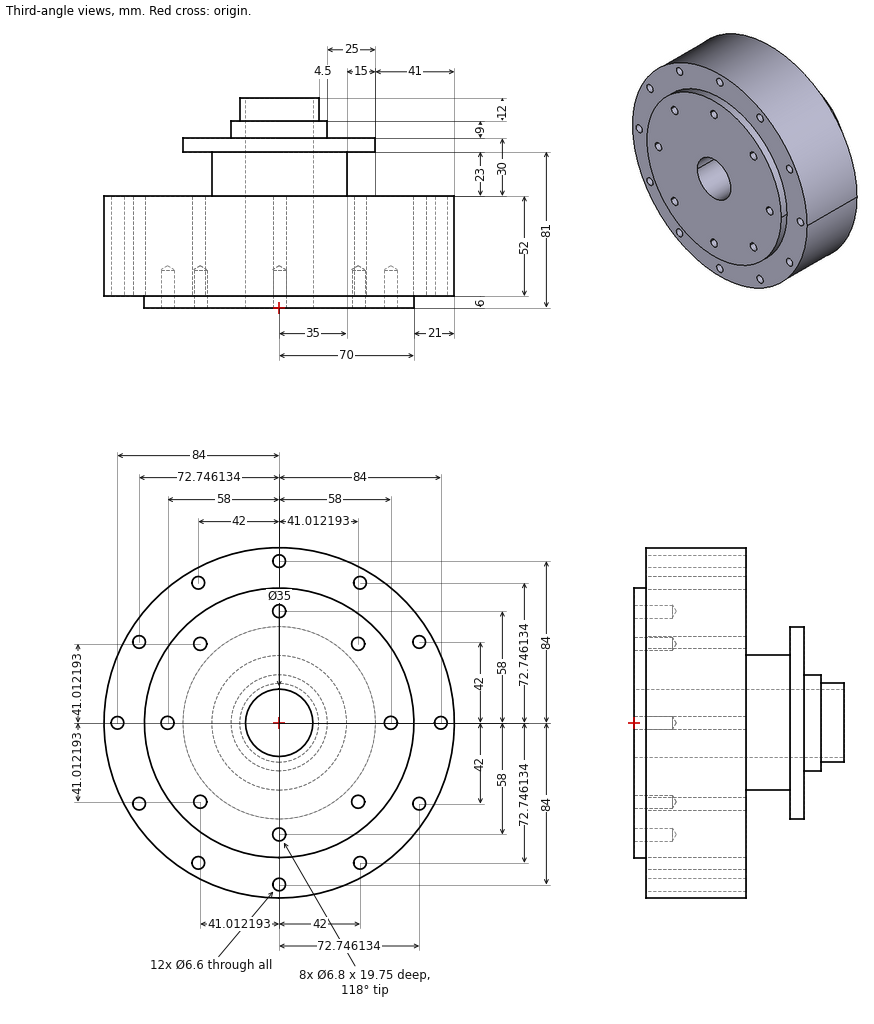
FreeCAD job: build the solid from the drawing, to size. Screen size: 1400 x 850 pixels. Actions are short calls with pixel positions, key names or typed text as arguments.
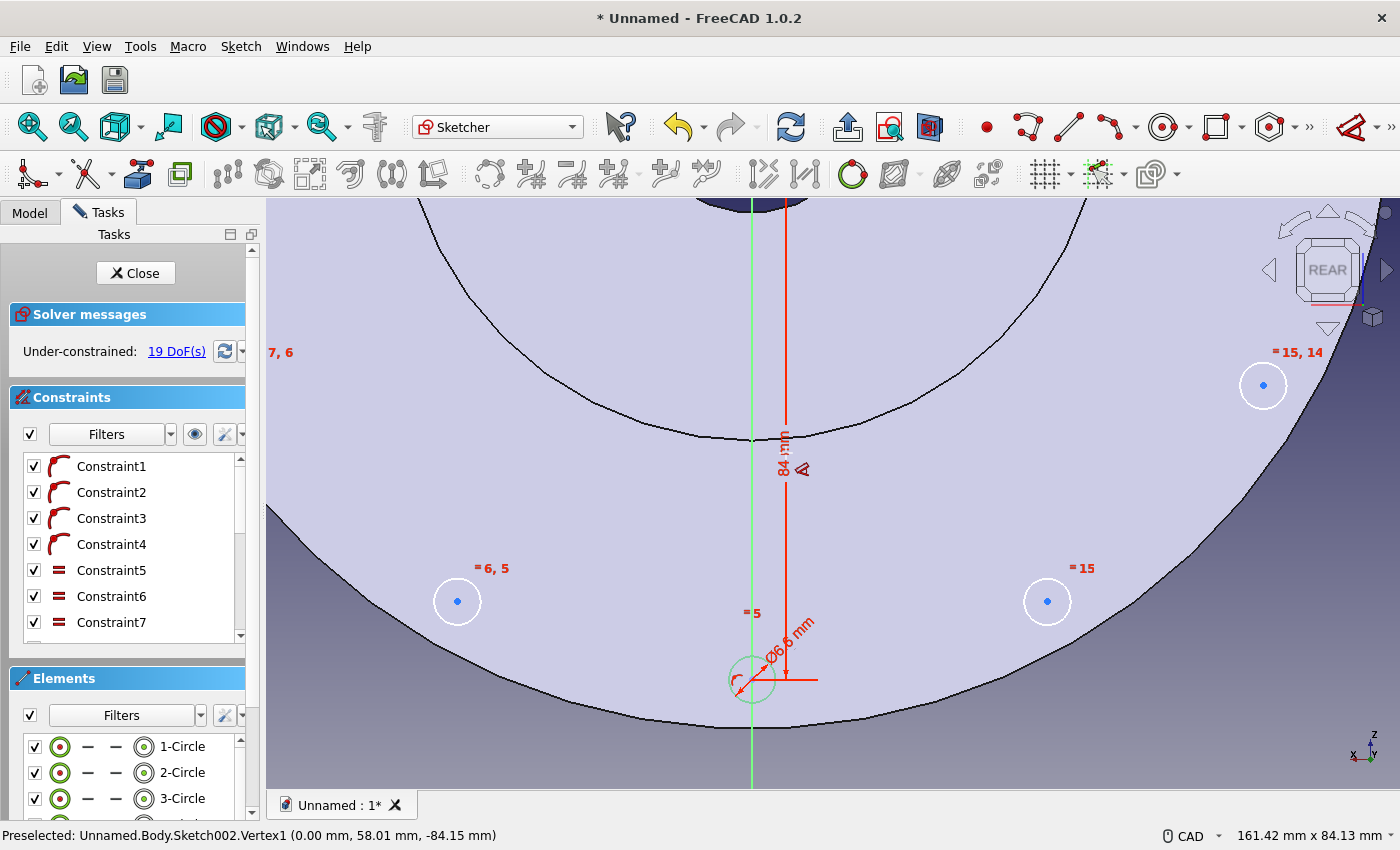
click(457, 602)
click(605, 636)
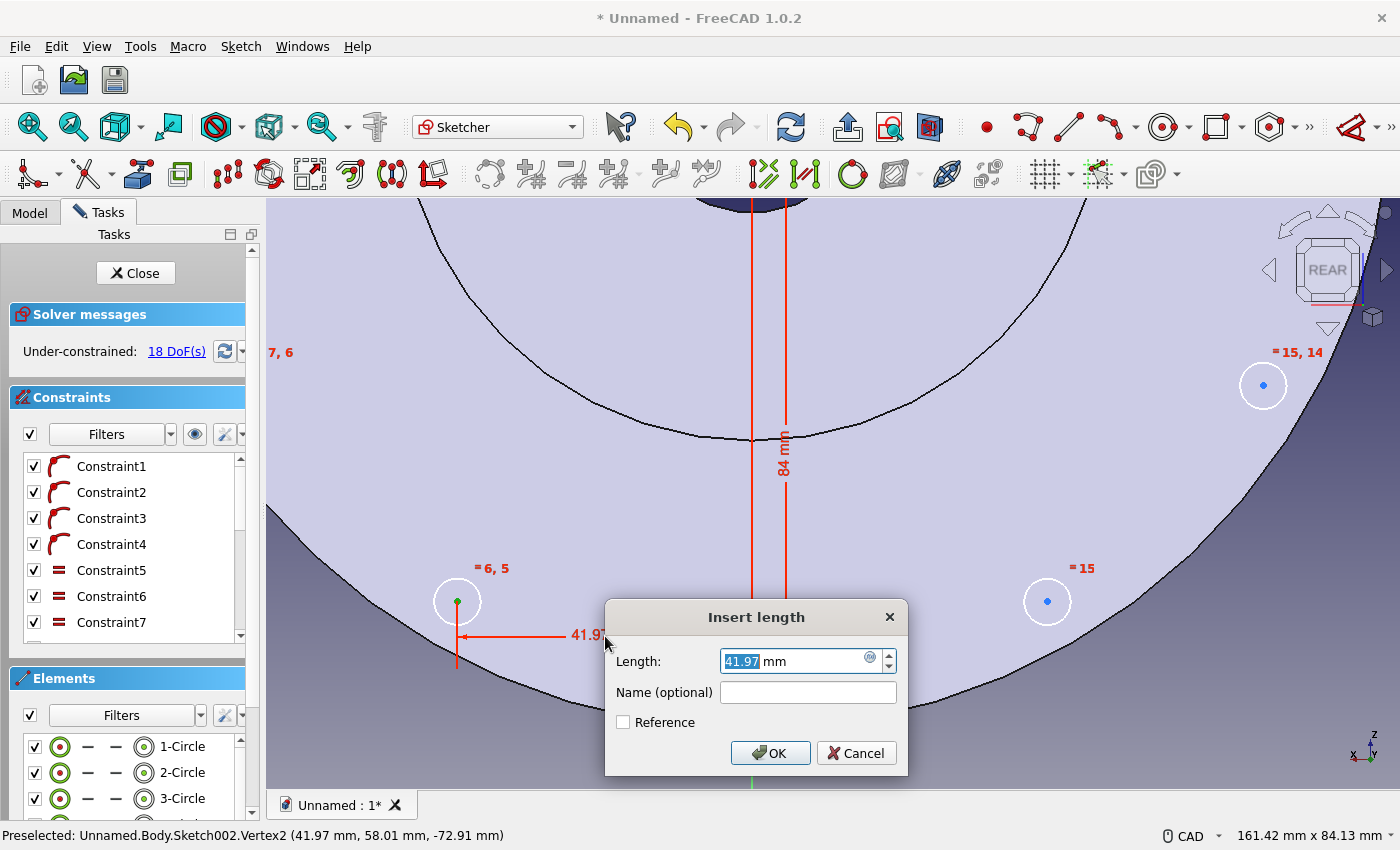
text(42)
key(Return)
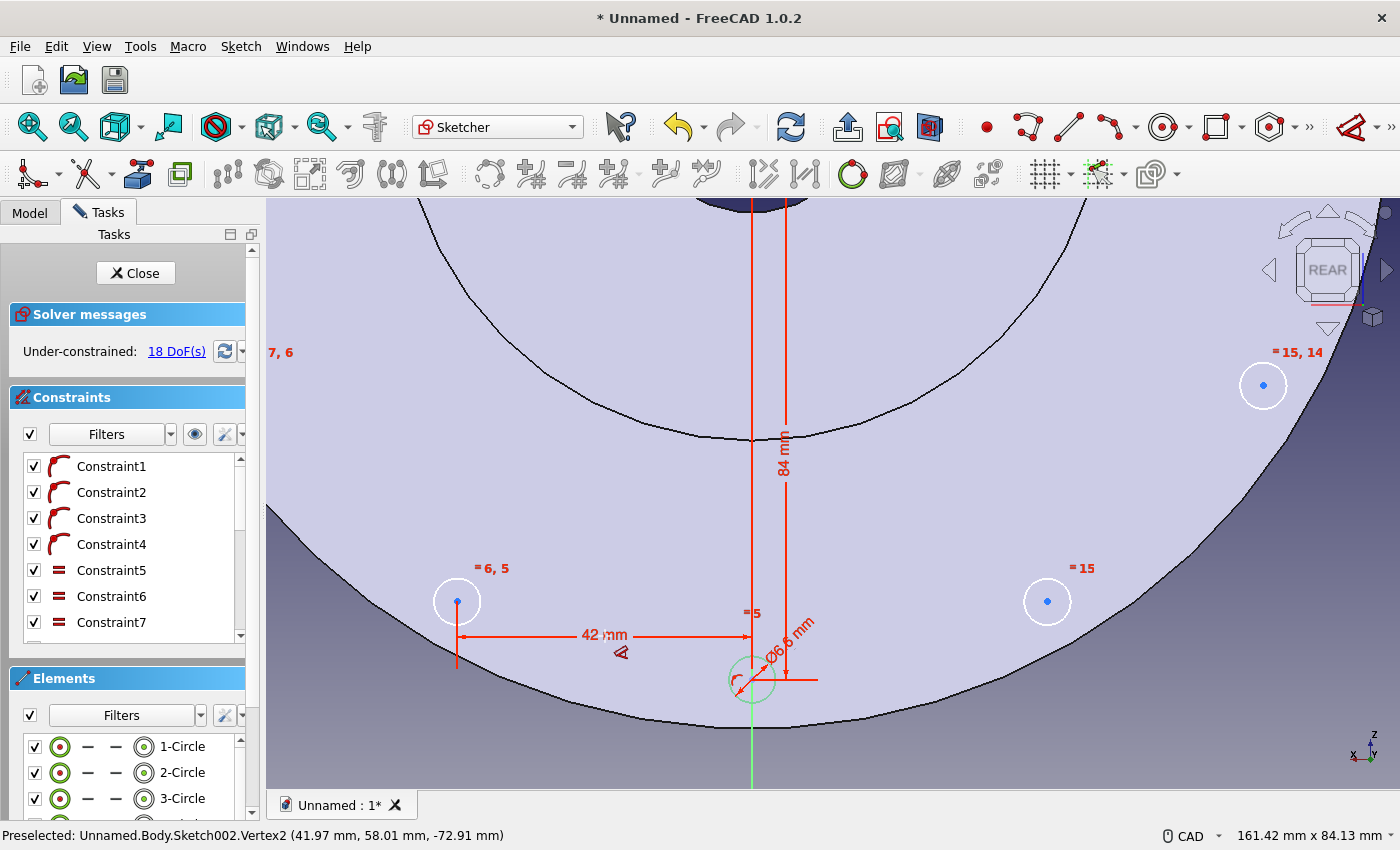
scroll(770, 668, down, 6)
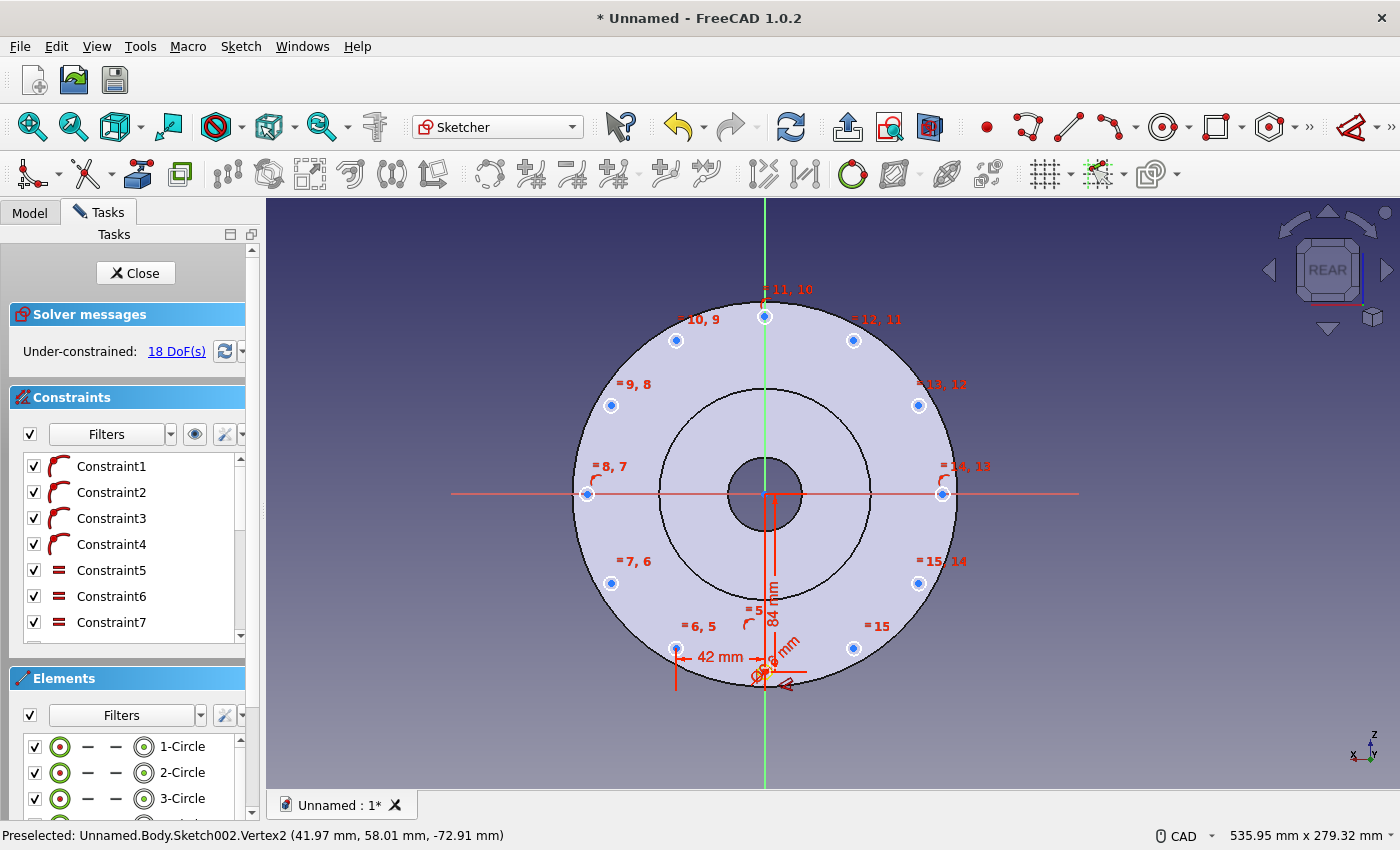
click(611, 584)
click(577, 539)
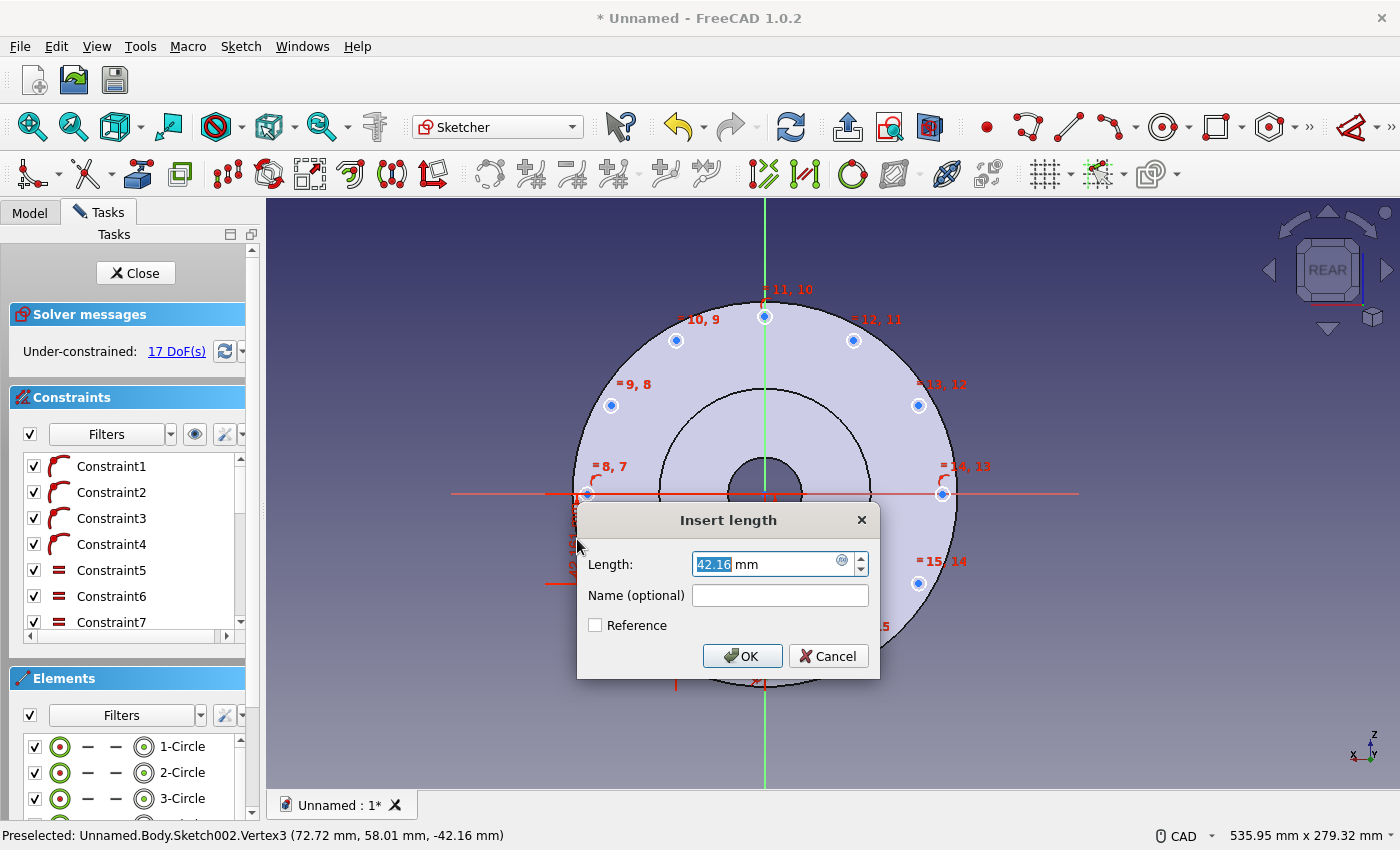
text(42)
key(Return)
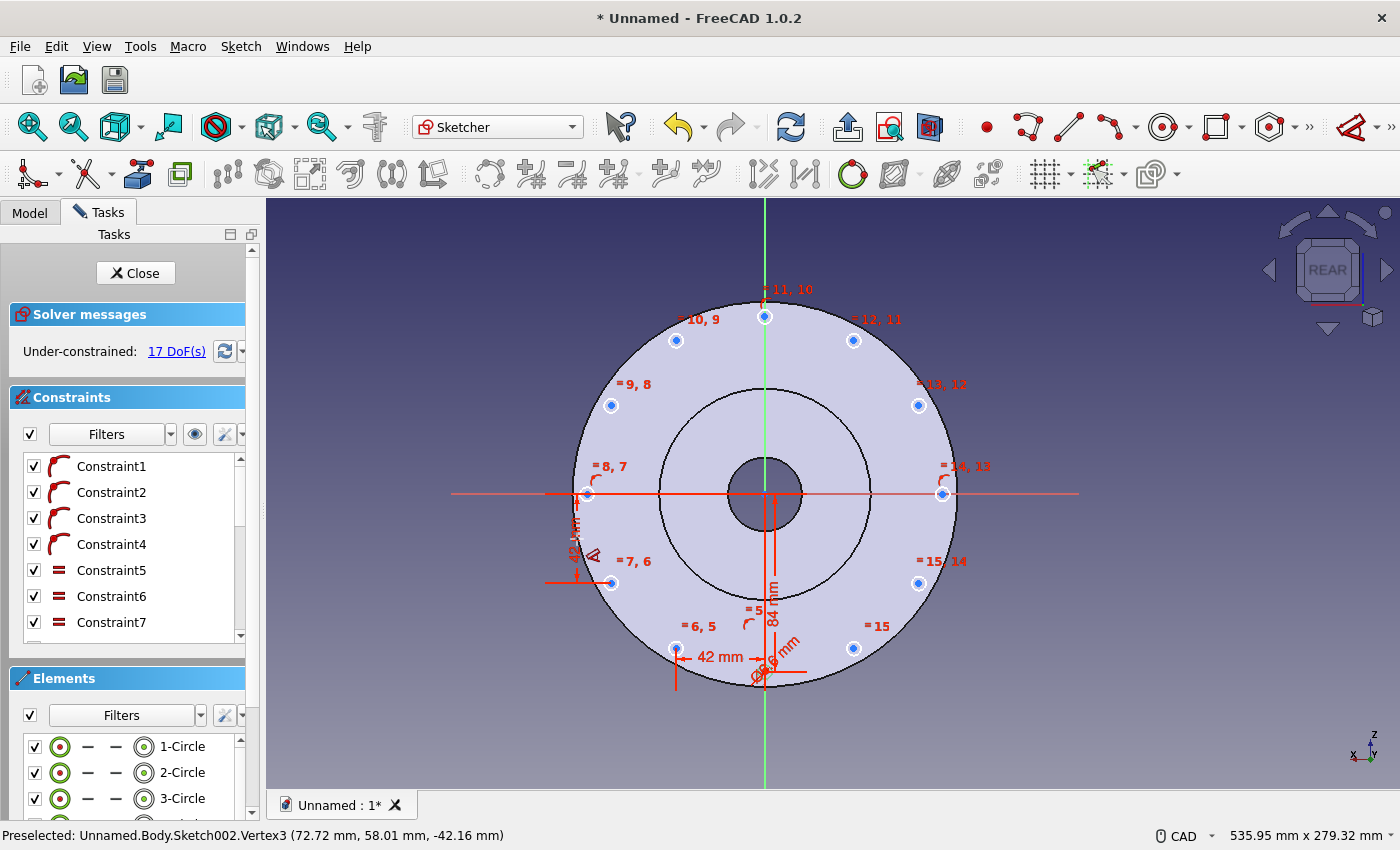
click(587, 494)
click(676, 528)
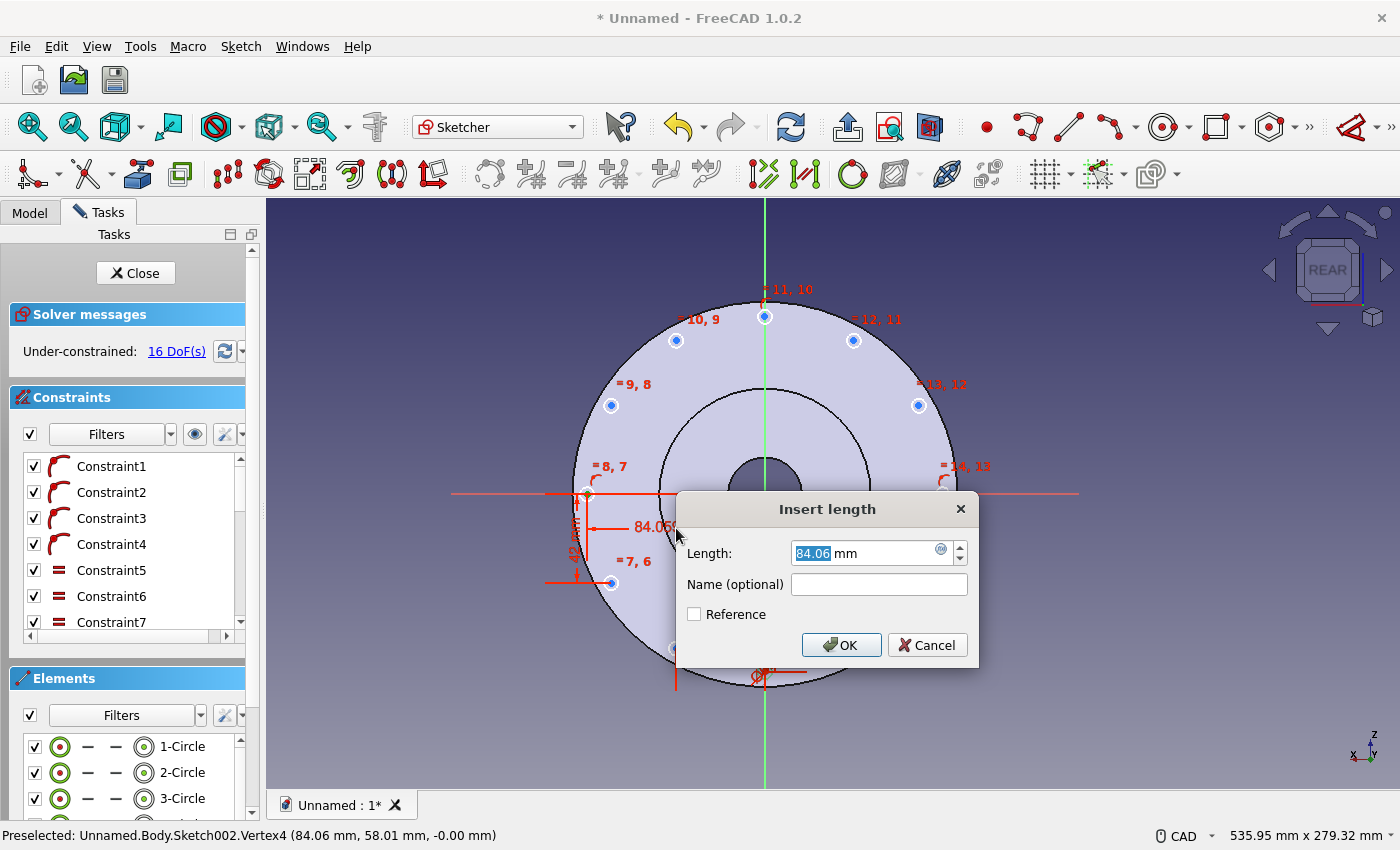
text(84)
key(Return)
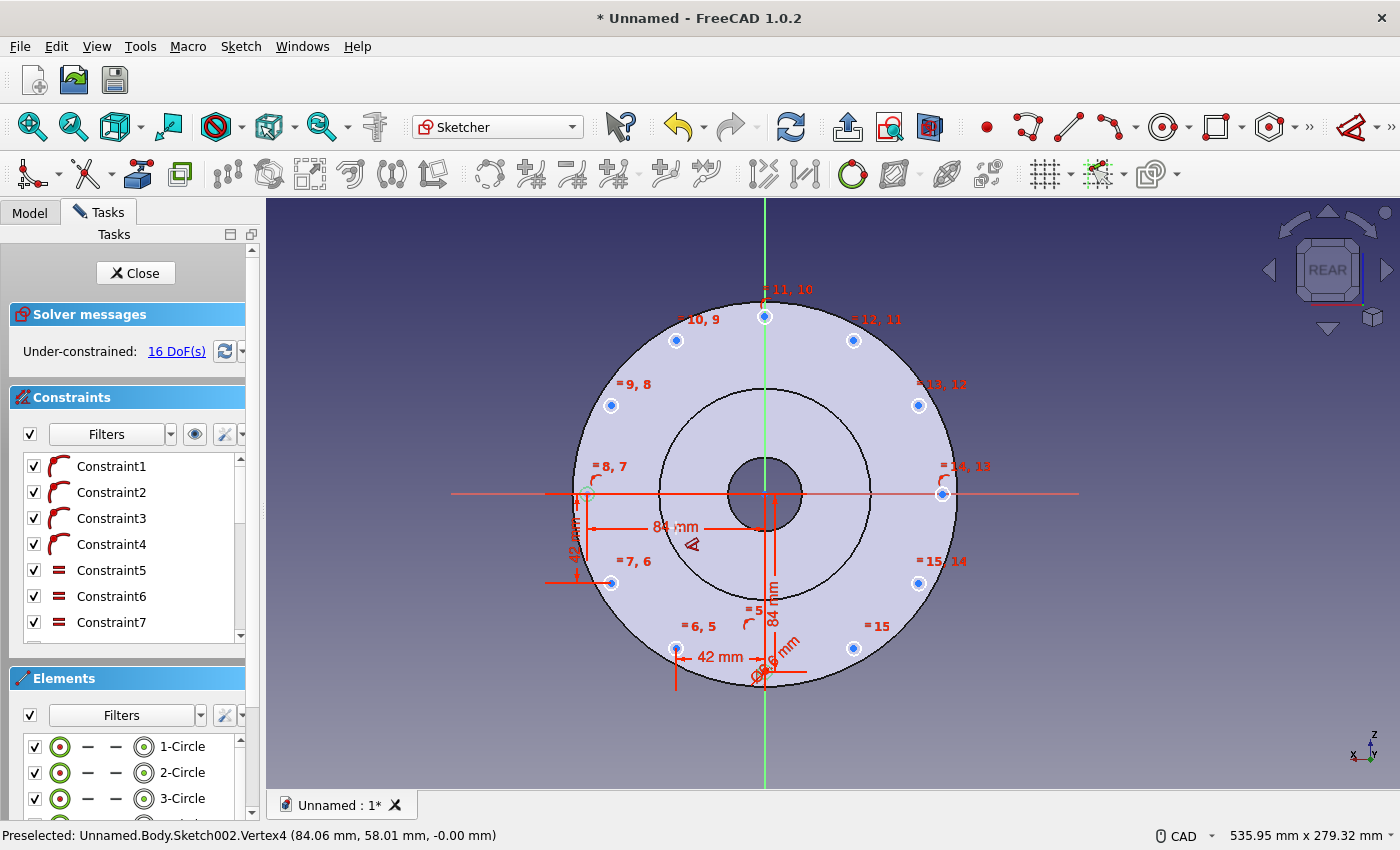
click(611, 406)
click(577, 450)